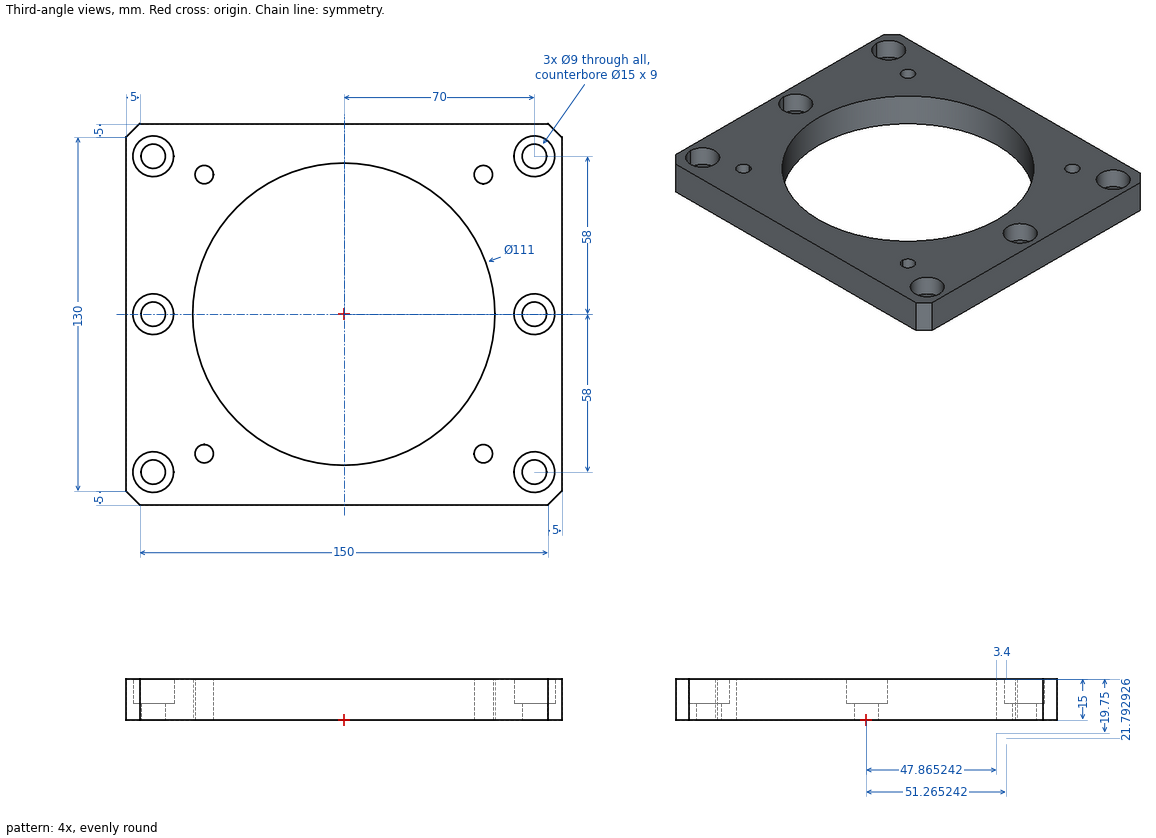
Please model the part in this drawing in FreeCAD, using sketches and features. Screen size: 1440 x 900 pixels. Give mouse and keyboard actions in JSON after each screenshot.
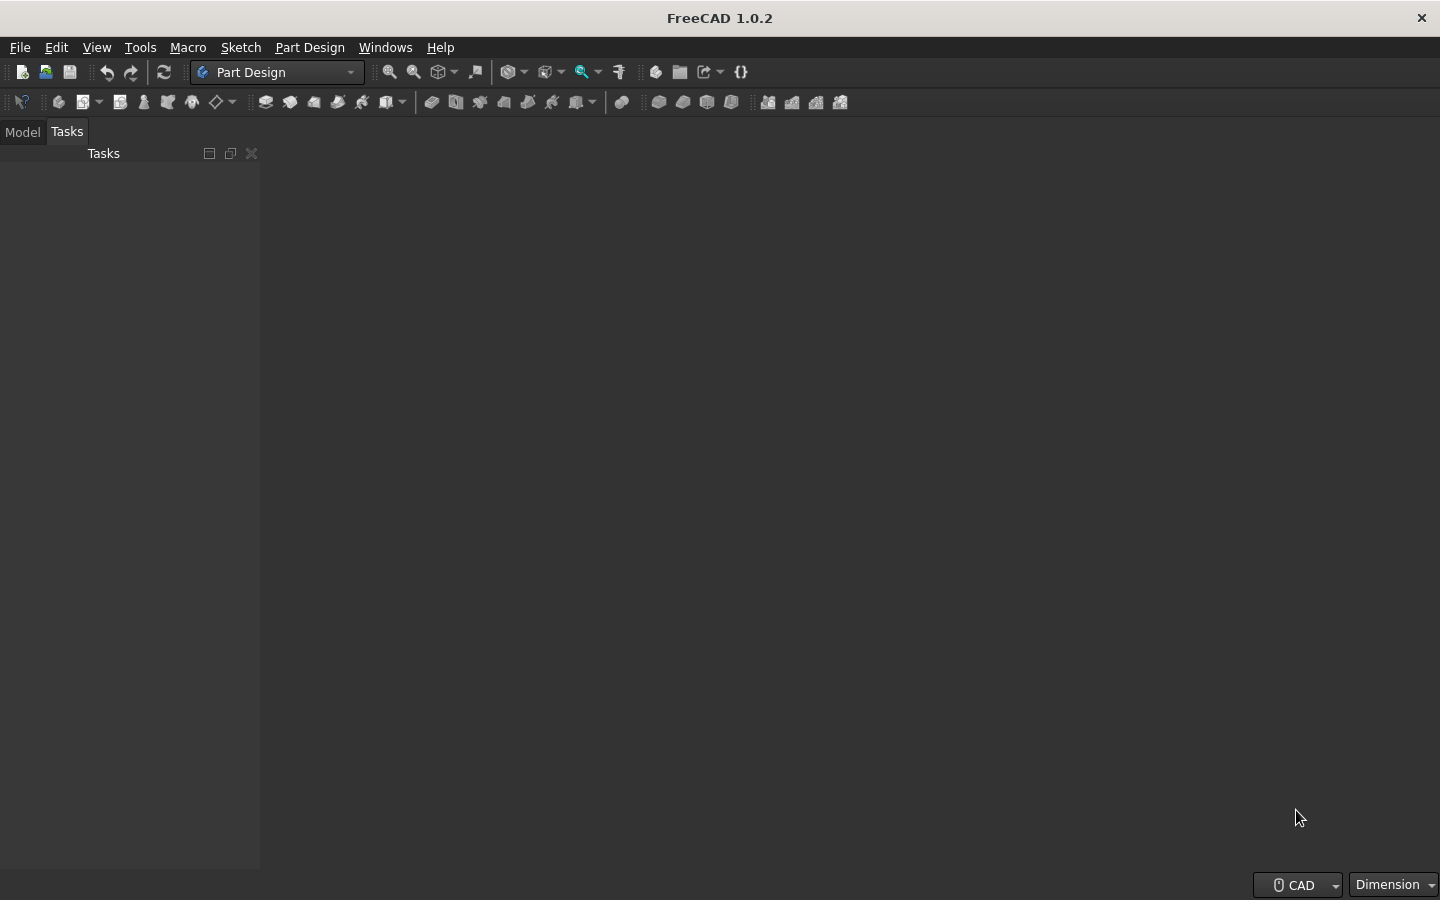
{"action": "left_click", "coordinate": [22, 72]}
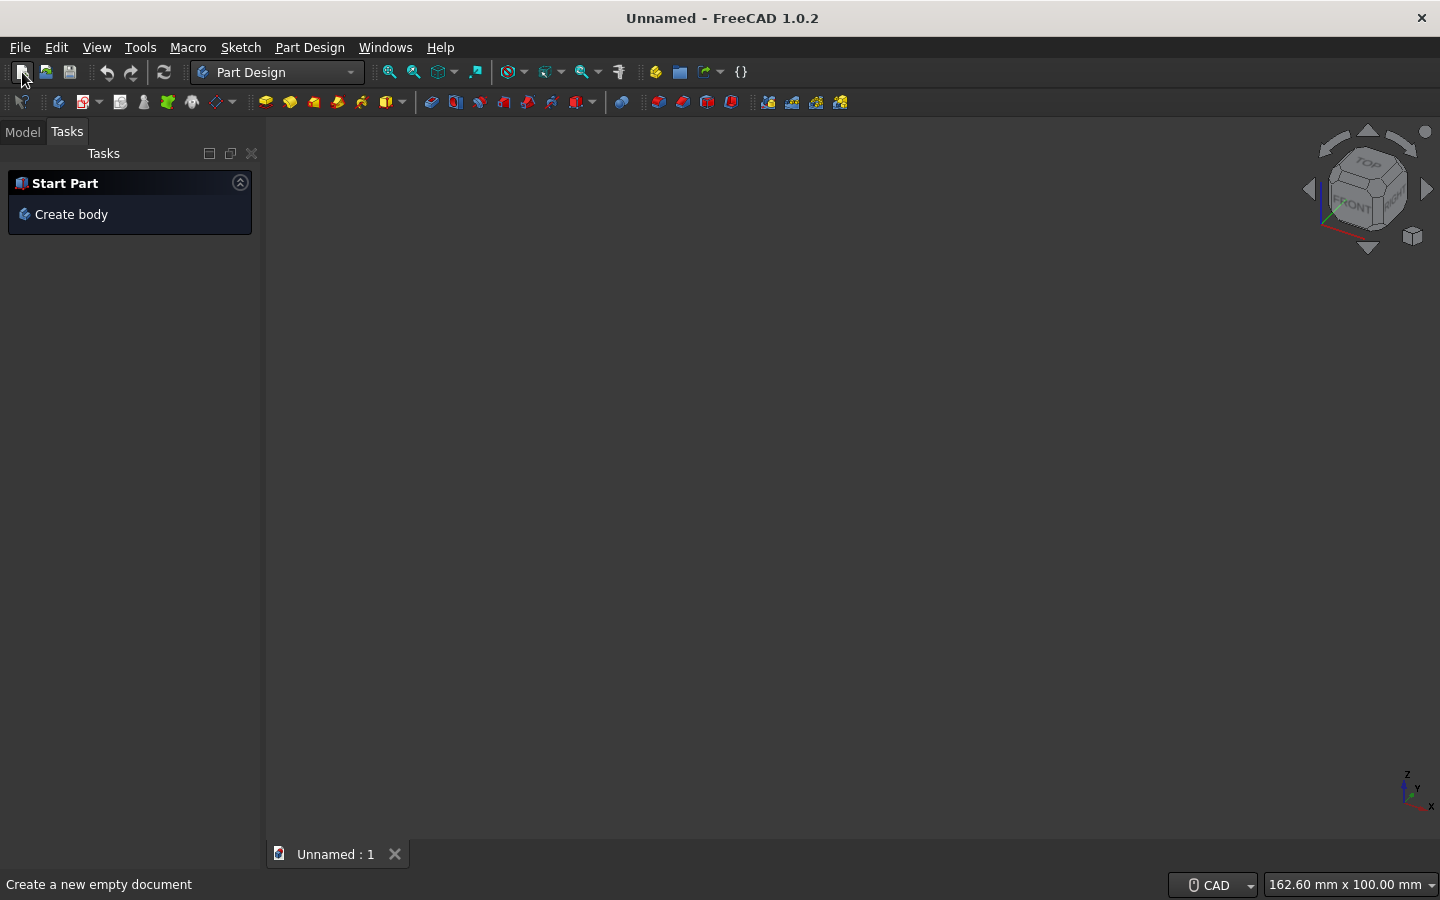
{"action": "left_click", "coordinate": [84, 102]}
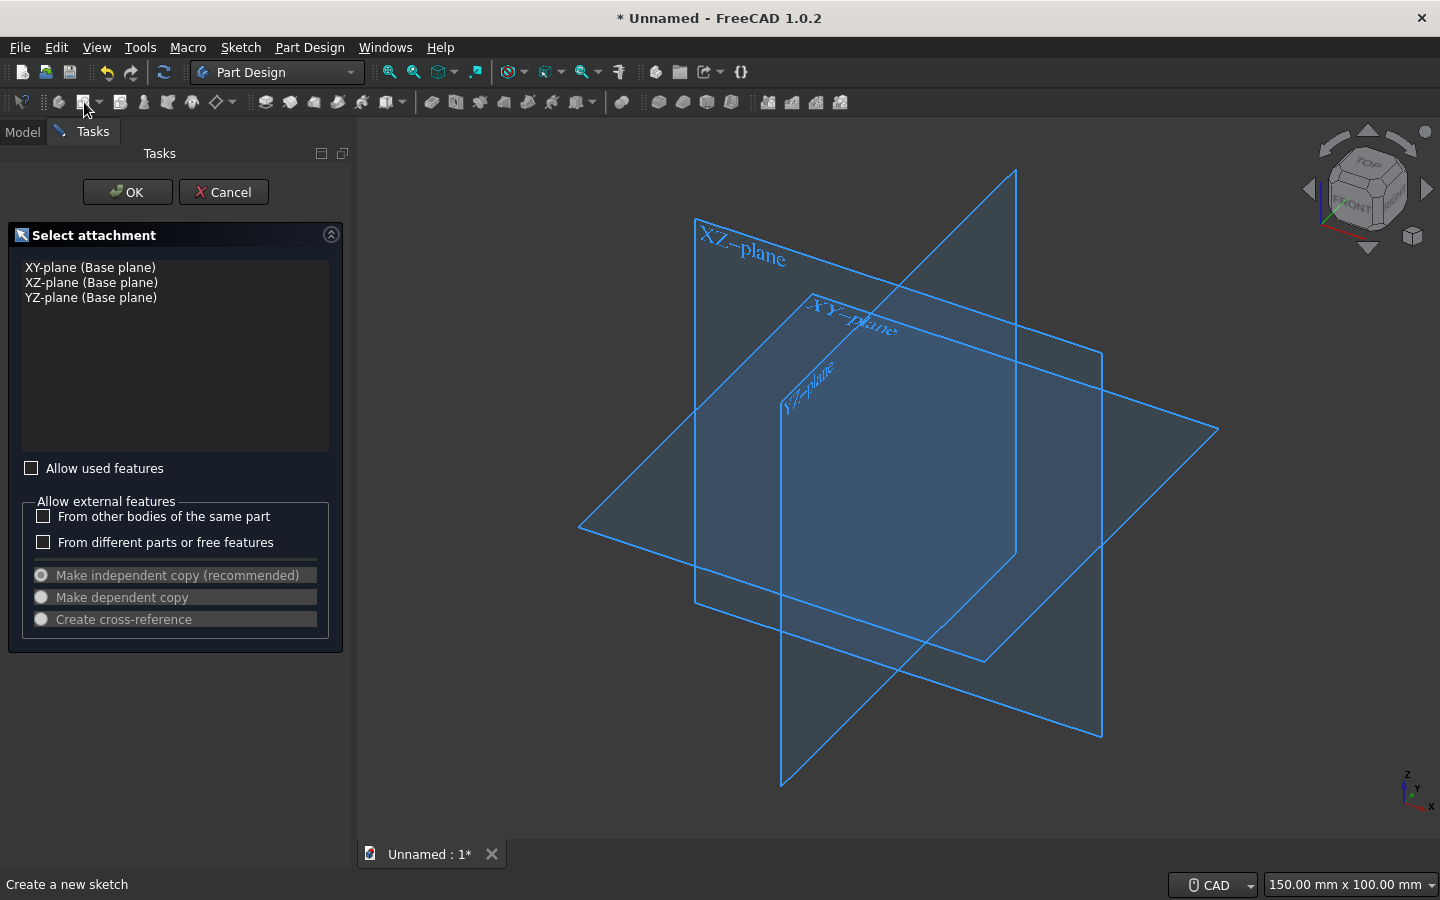
{"action": "left_click", "coordinate": [82, 268]}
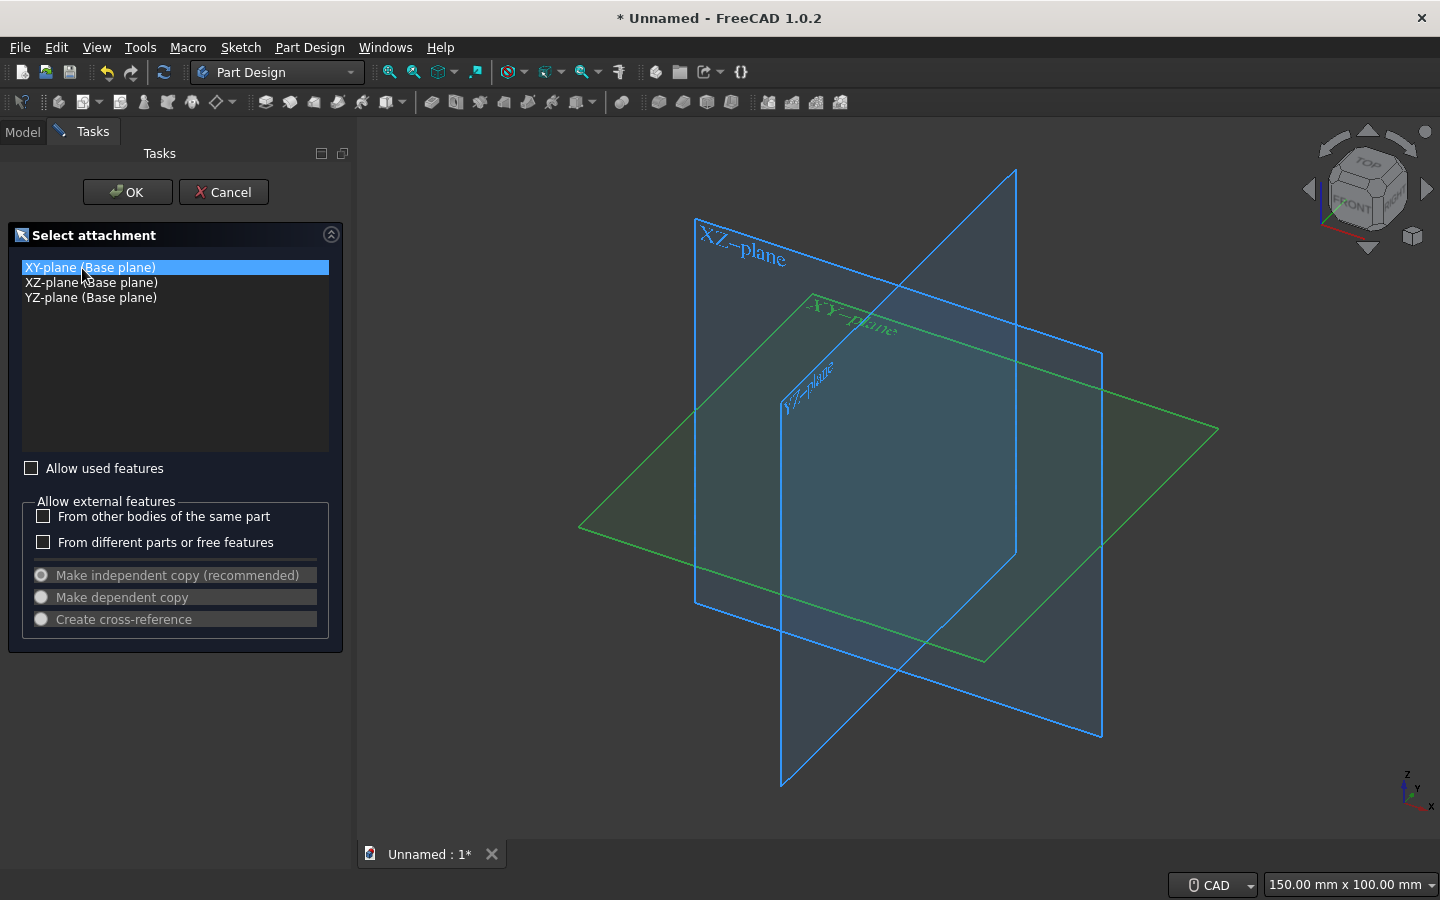
{"action": "left_click", "coordinate": [128, 192]}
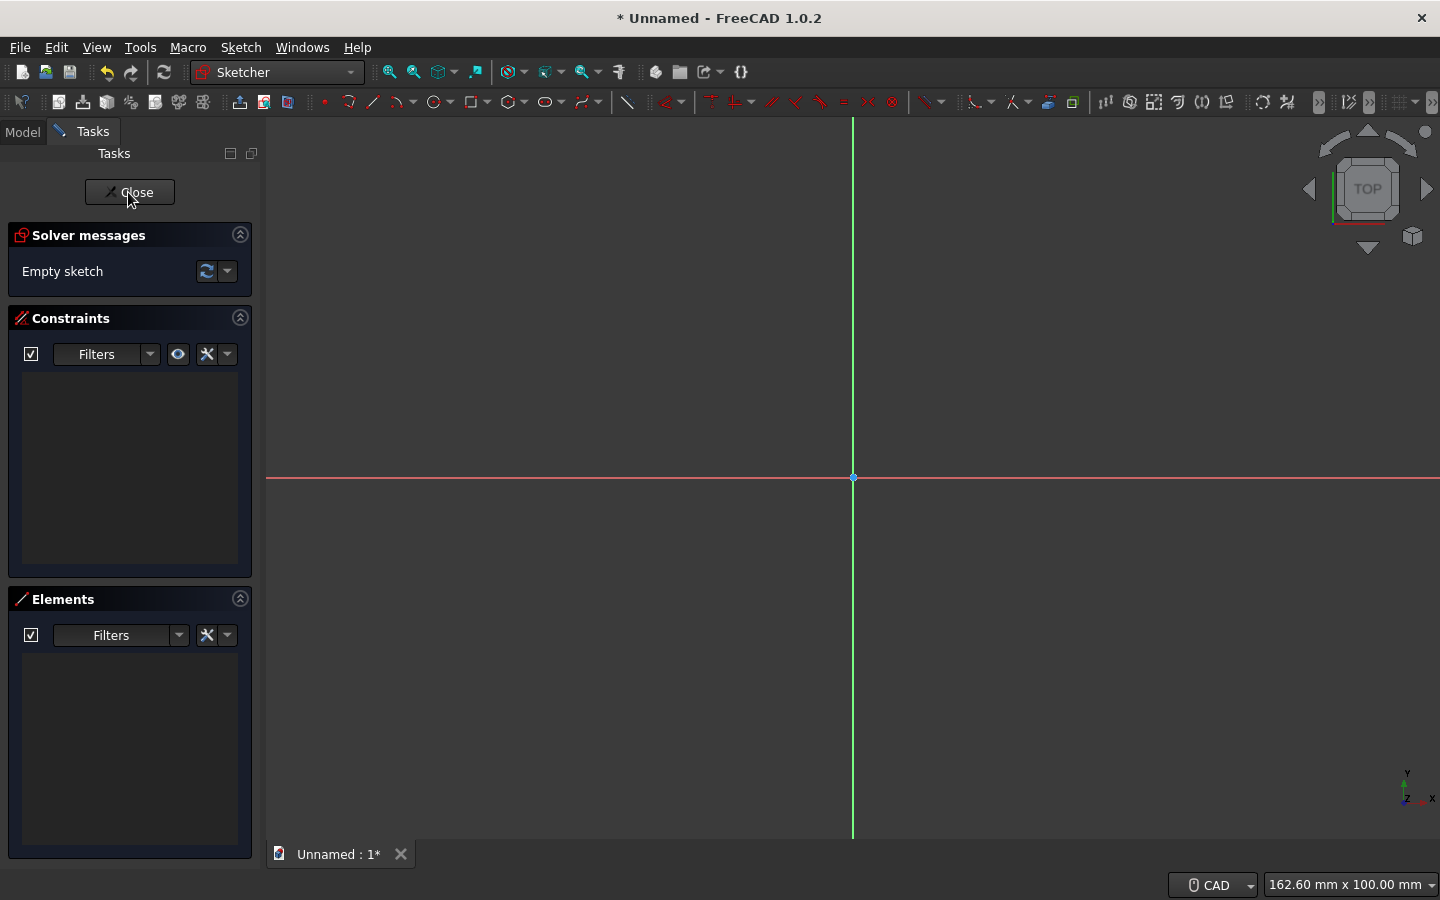
{"action": "scroll", "coordinate": [729, 478], "scroll_direction": "down", "scroll_amount": 4}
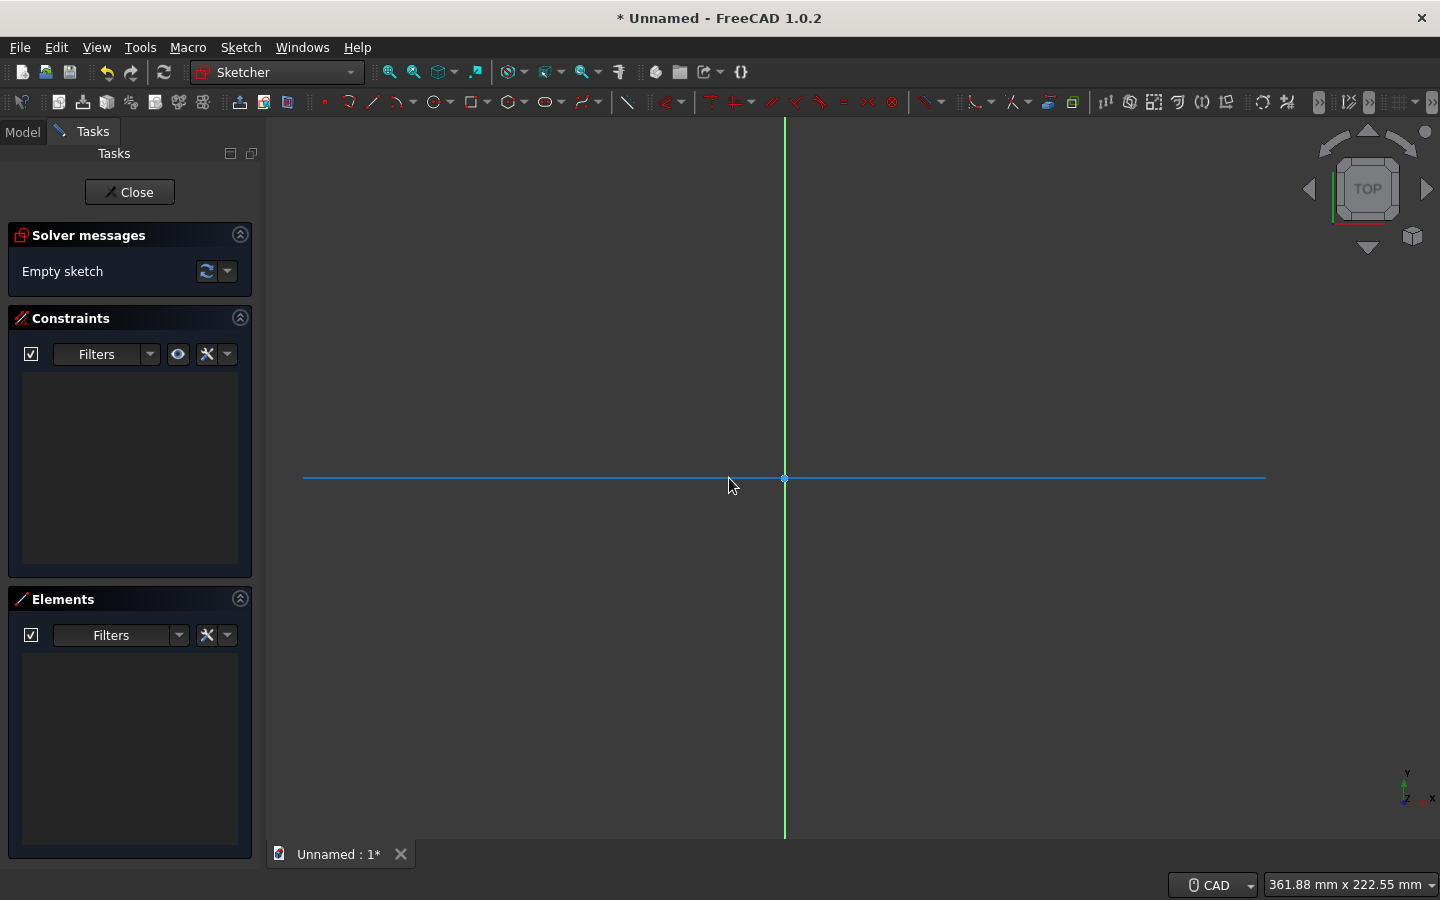
{"action": "left_click", "coordinate": [350, 102]}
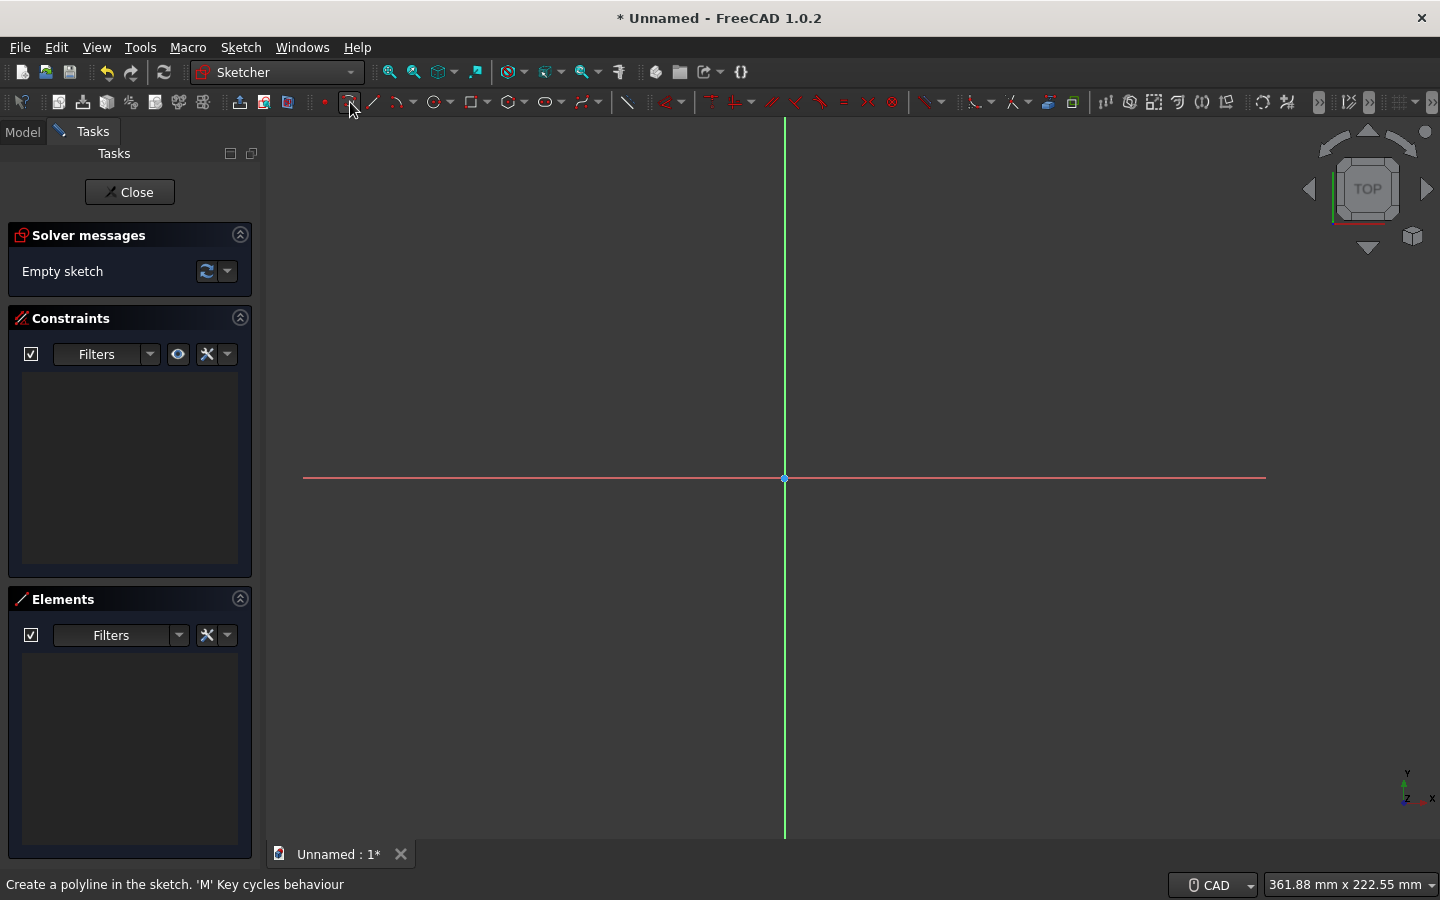
{"action": "left_click", "coordinate": [542, 251]}
{"action": "left_click", "coordinate": [525, 267]}
{"action": "left_click", "coordinate": [525, 689]}
{"action": "left_click", "coordinate": [542, 705]}
{"action": "left_click", "coordinate": [1028, 705]}
{"action": "left_click", "coordinate": [1044, 689]}
{"action": "left_click", "coordinate": [1044, 267]}
{"action": "left_click", "coordinate": [1028, 251]}